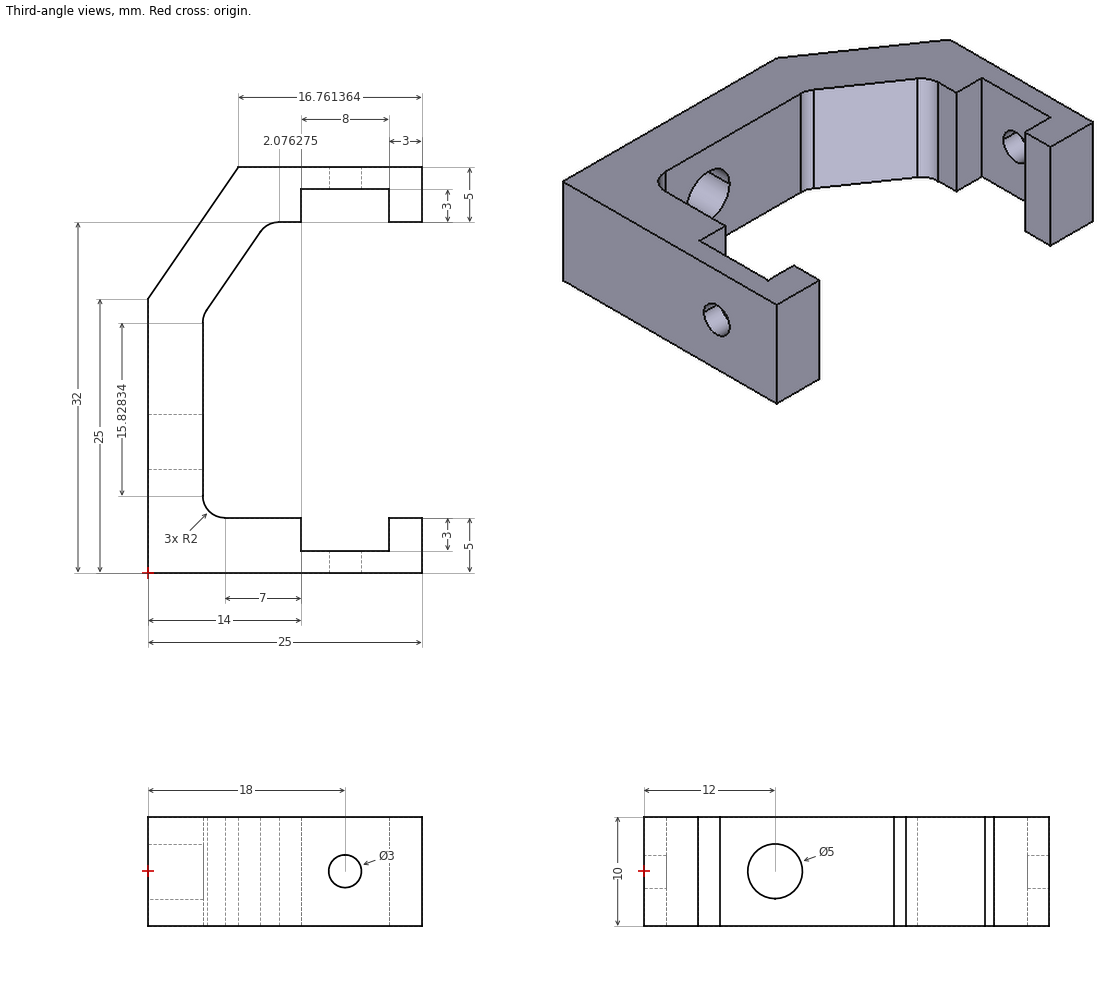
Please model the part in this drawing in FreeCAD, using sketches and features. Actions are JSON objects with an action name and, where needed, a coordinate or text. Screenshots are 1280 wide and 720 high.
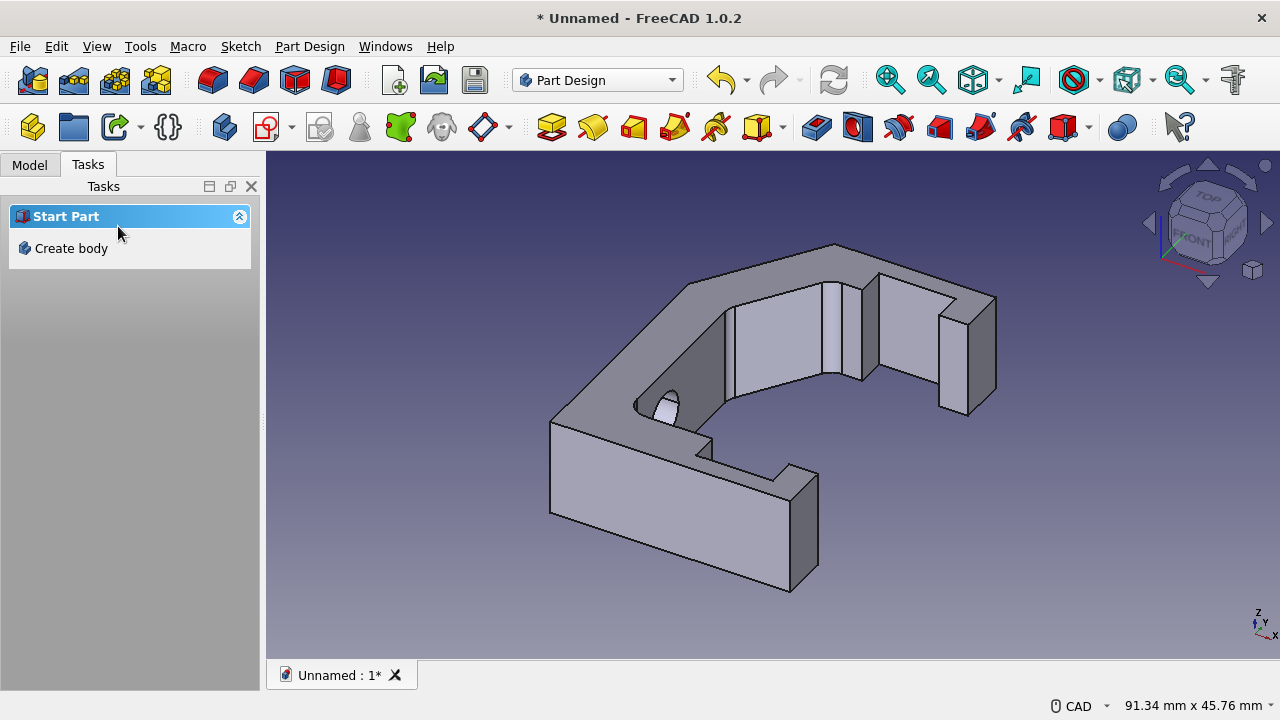
{"action": "key", "text": "4"}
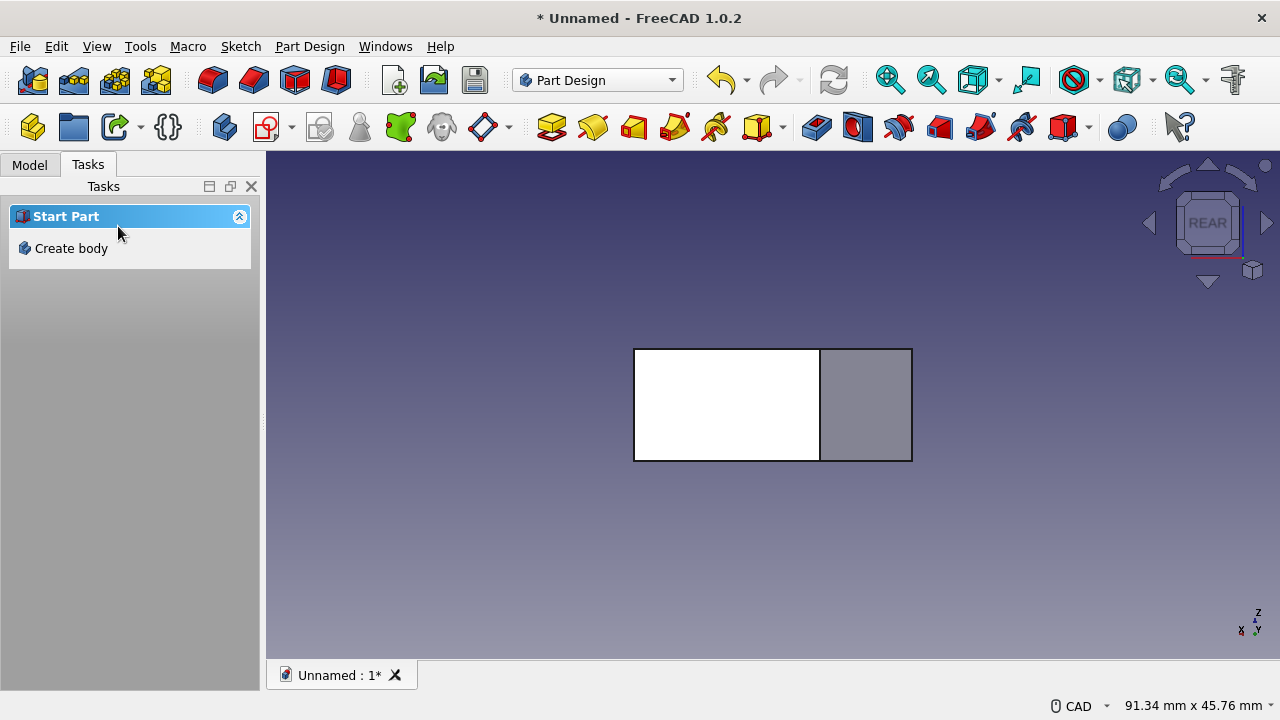
{"action": "left_click", "coordinate": [891, 80]}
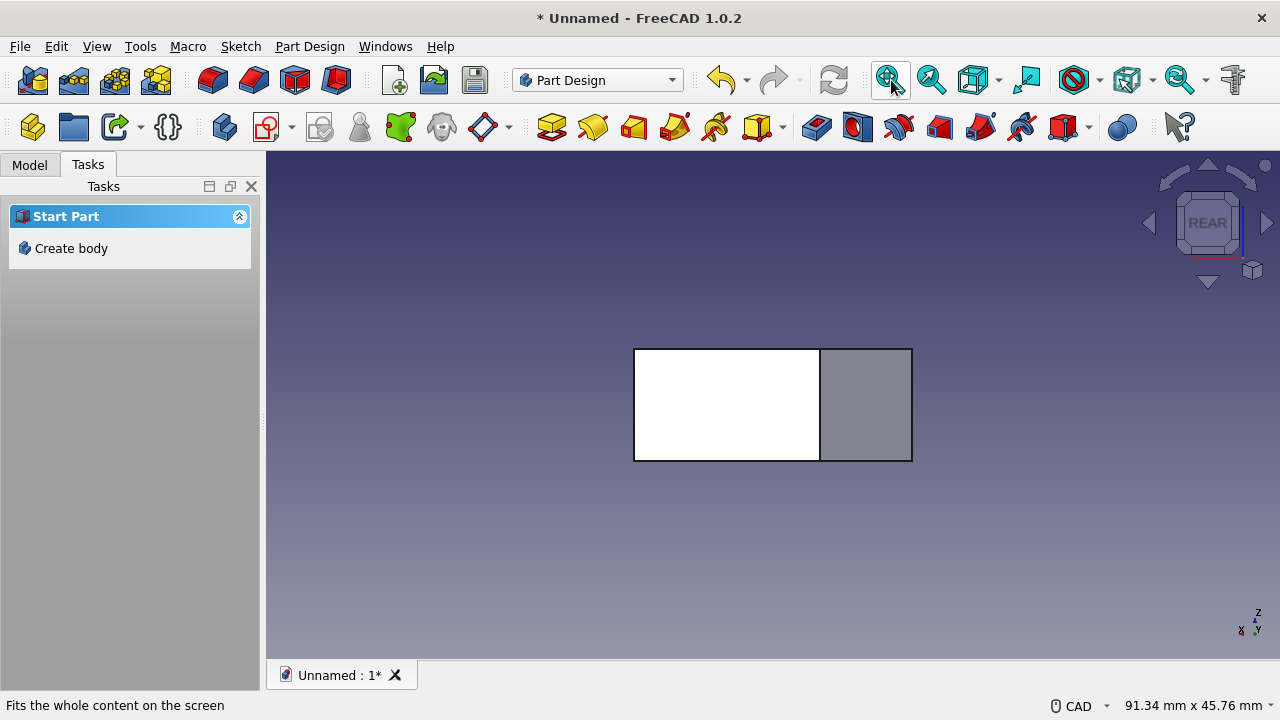
{"action": "left_click", "coordinate": [701, 404]}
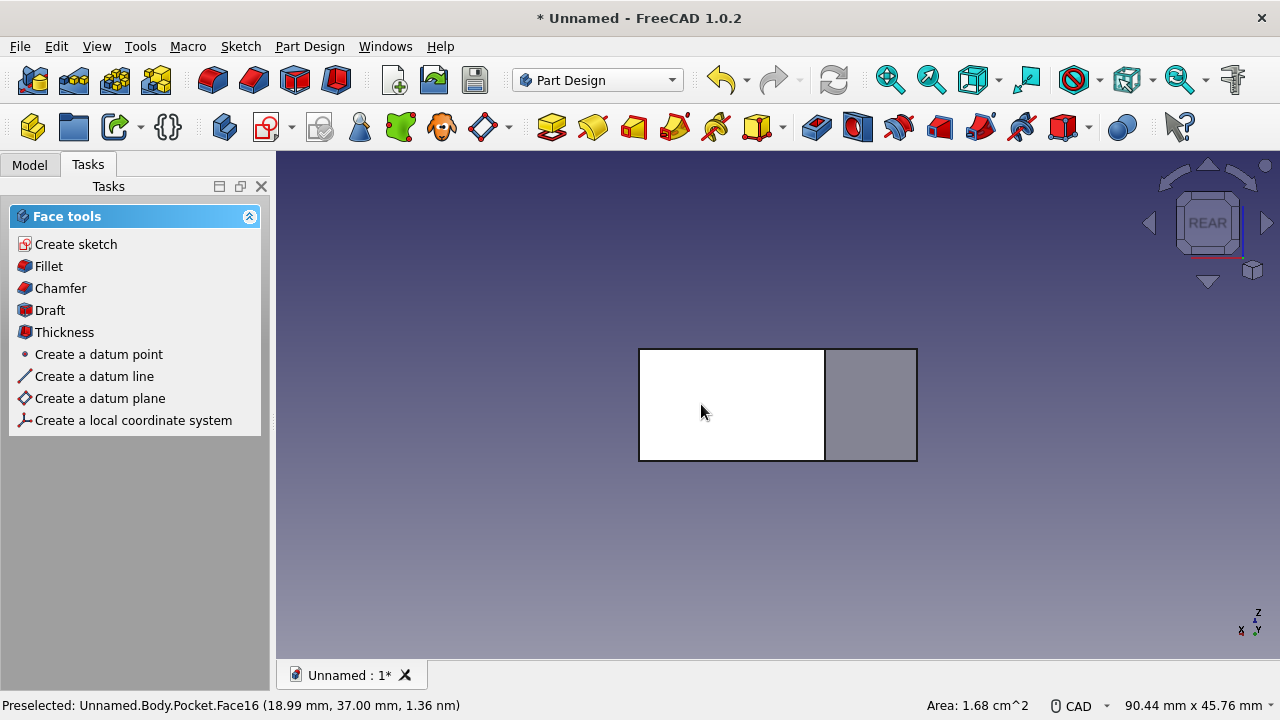
{"action": "left_click", "coordinate": [266, 128]}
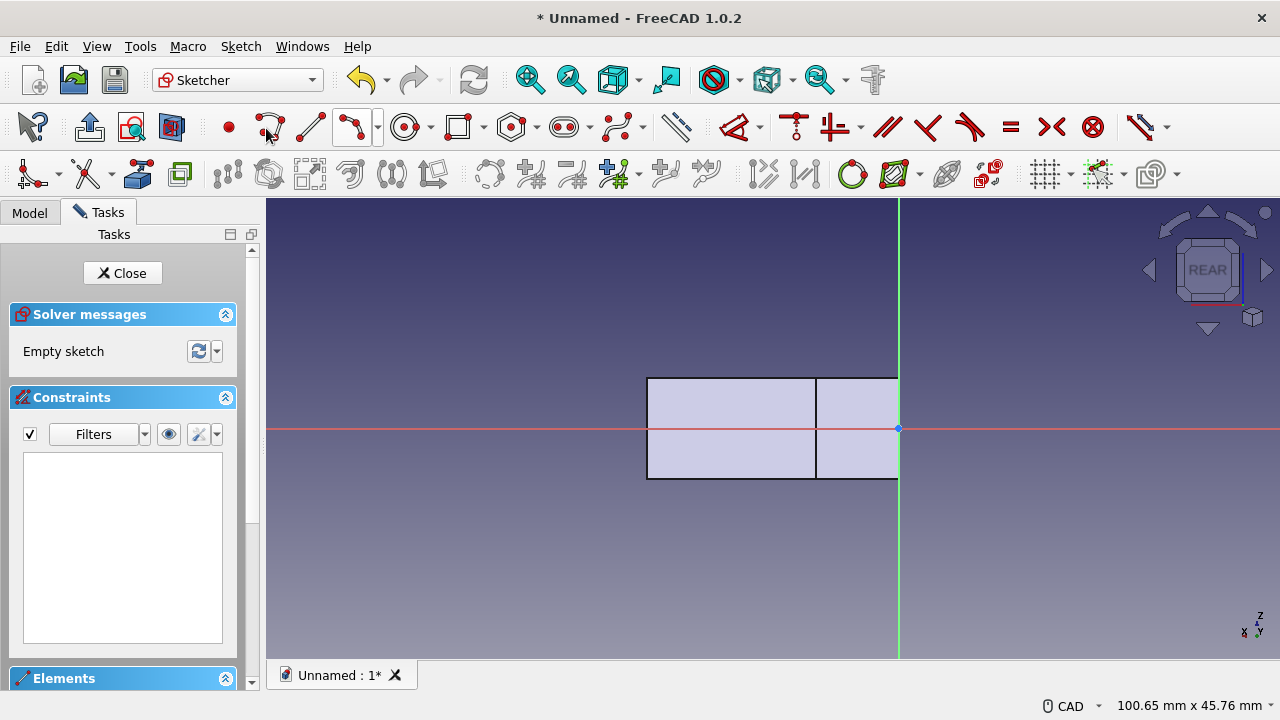
{"action": "scroll", "coordinate": [719, 428], "scroll_direction": "up", "scroll_amount": 11}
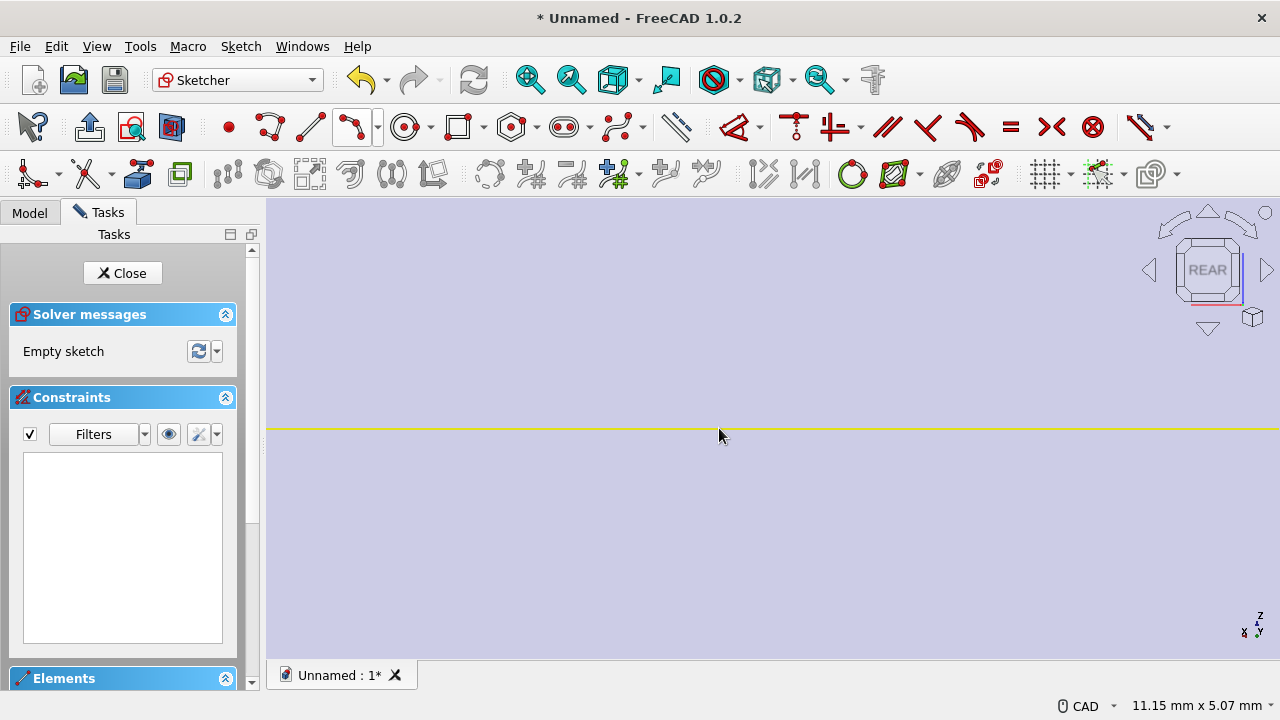
{"action": "left_click", "coordinate": [404, 128]}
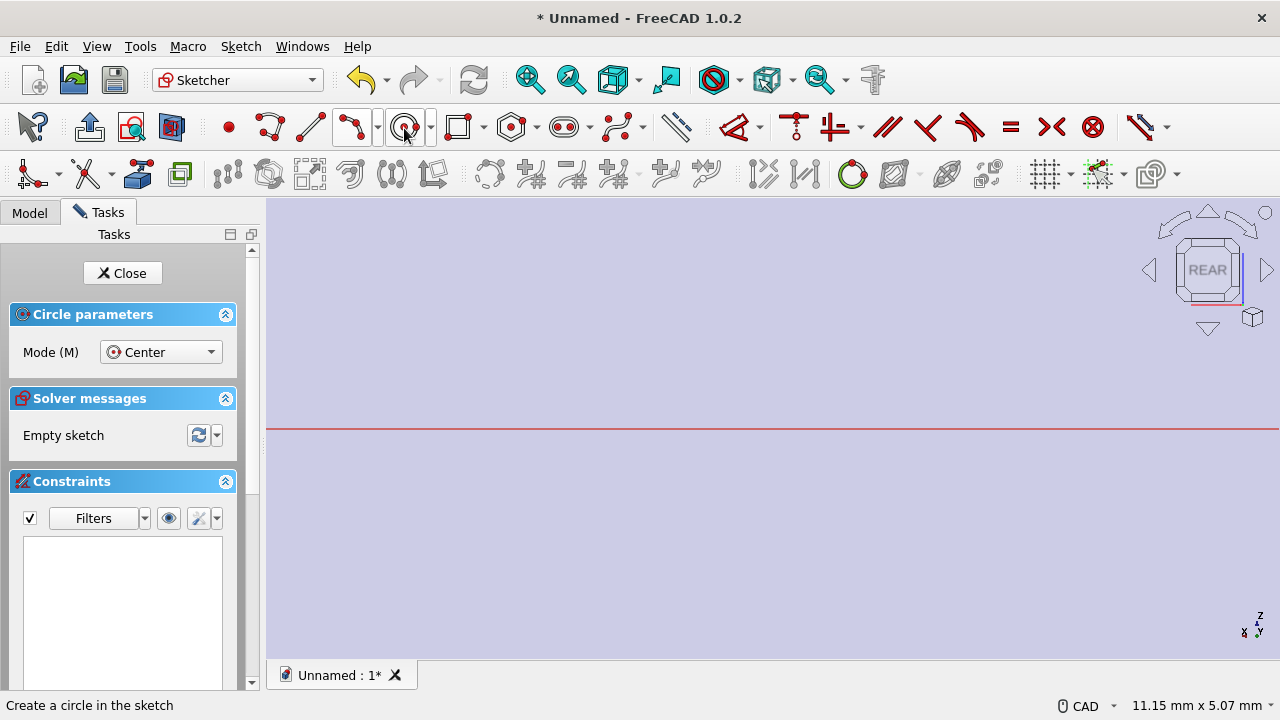
{"action": "left_click", "coordinate": [703, 428]}
{"action": "mouse_move", "coordinate": [799, 332]}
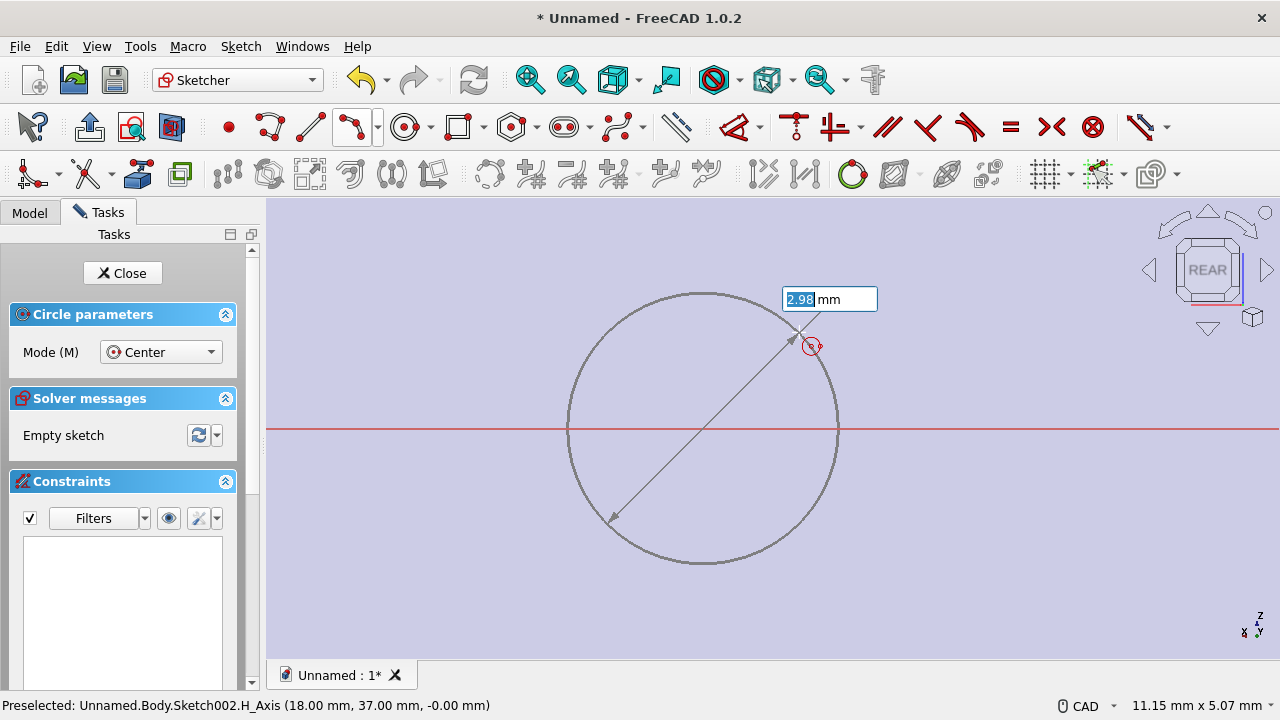
{"action": "type", "text": "3"}
{"action": "key", "text": "Return"}
{"action": "key", "text": "Escape"}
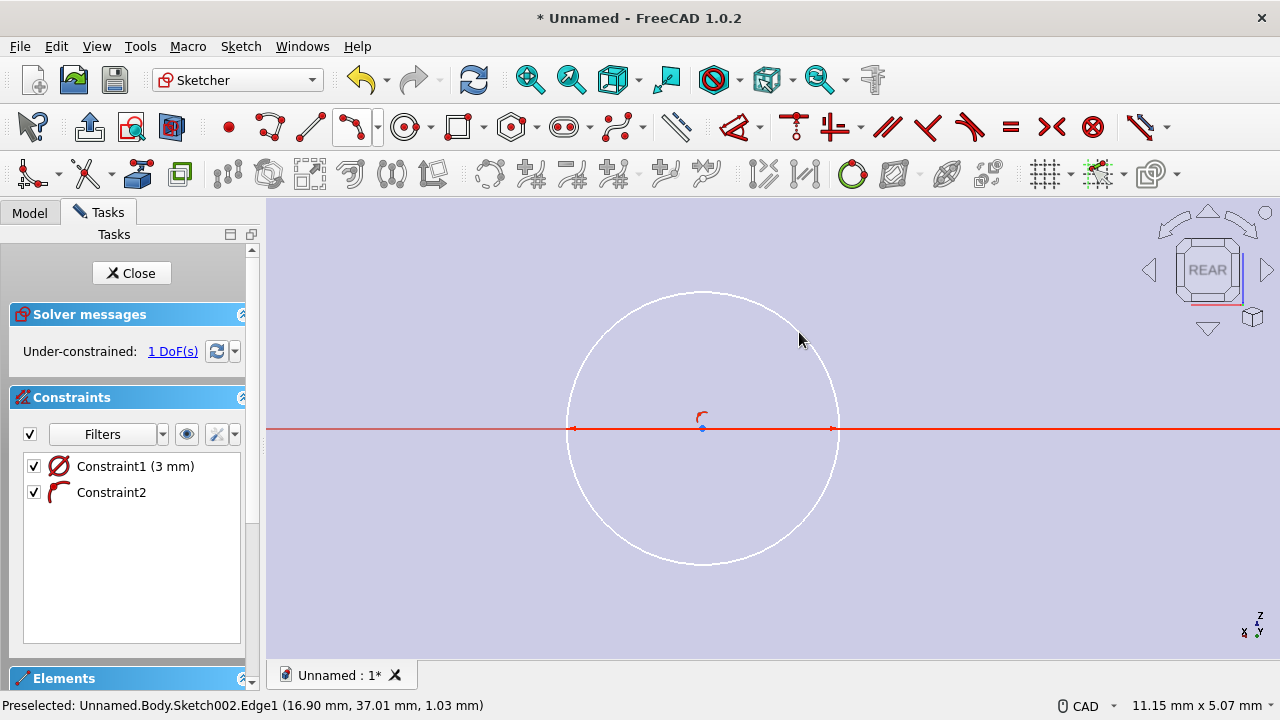
{"action": "left_click", "coordinate": [734, 128]}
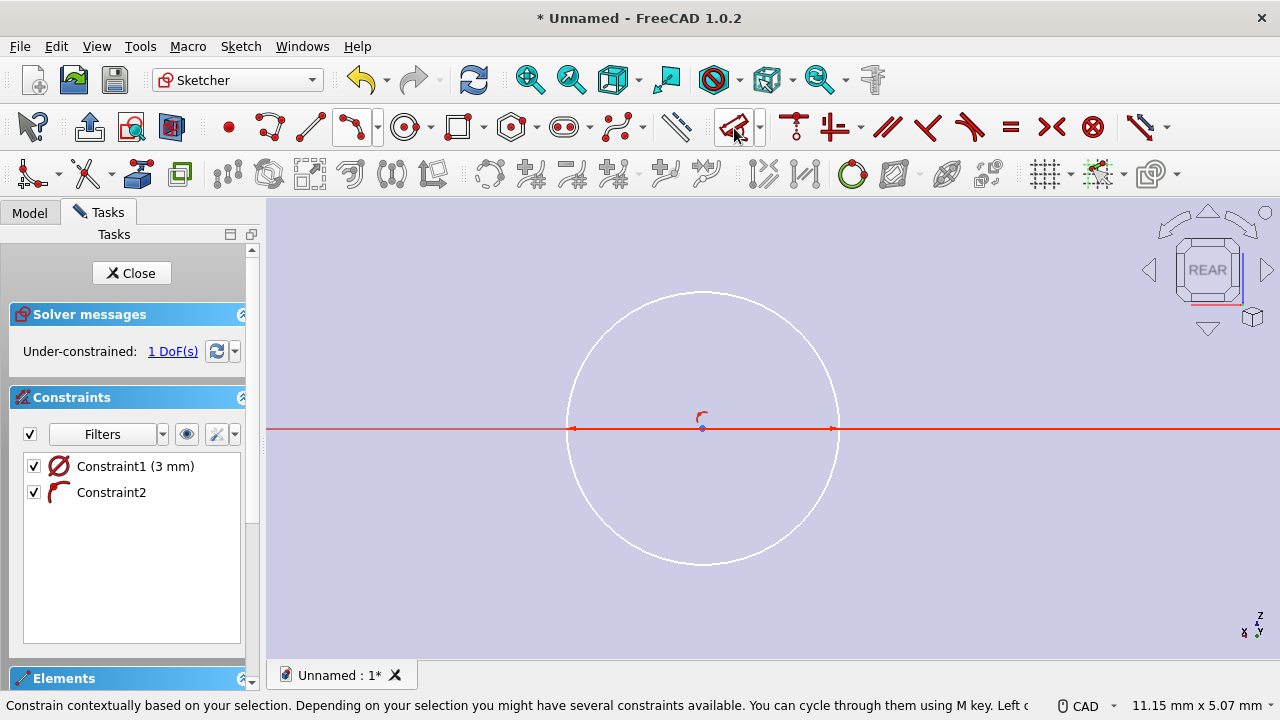
{"action": "left_click", "coordinate": [703, 428]}
{"action": "left_click", "coordinate": [909, 462]}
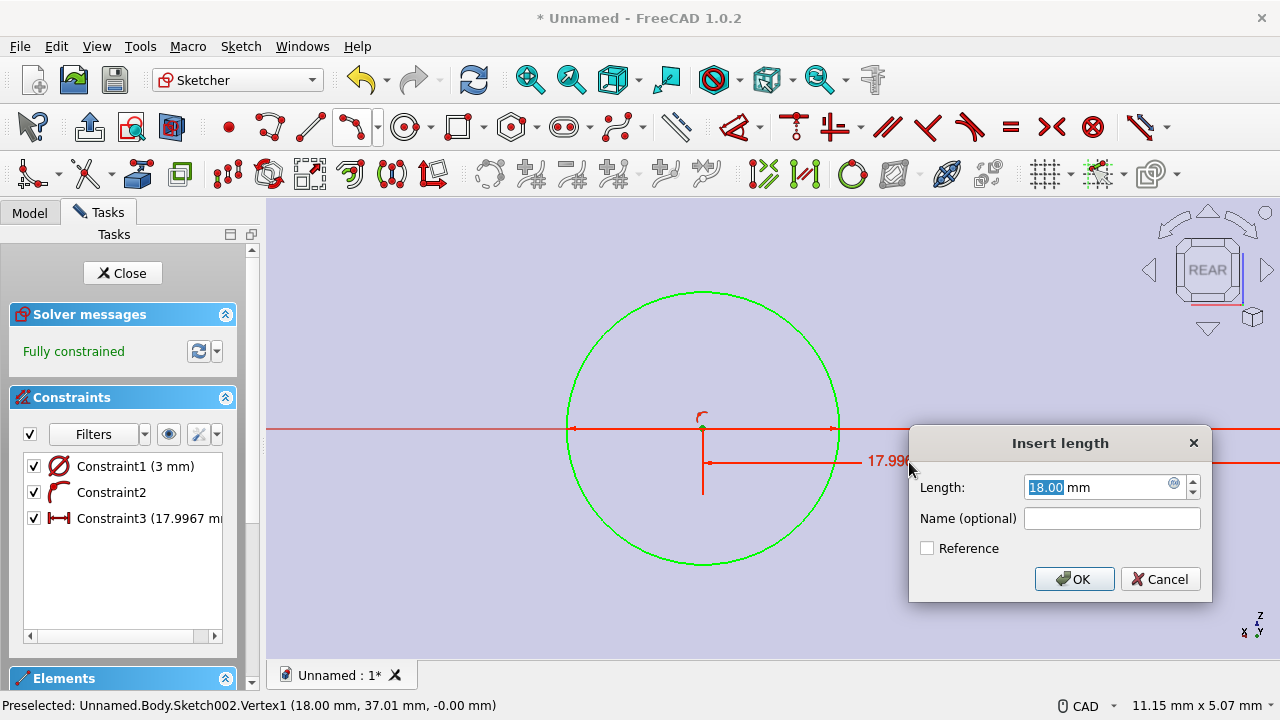
{"action": "type", "text": "18"}
{"action": "key", "text": "Return"}
{"action": "key", "text": "Escape"}